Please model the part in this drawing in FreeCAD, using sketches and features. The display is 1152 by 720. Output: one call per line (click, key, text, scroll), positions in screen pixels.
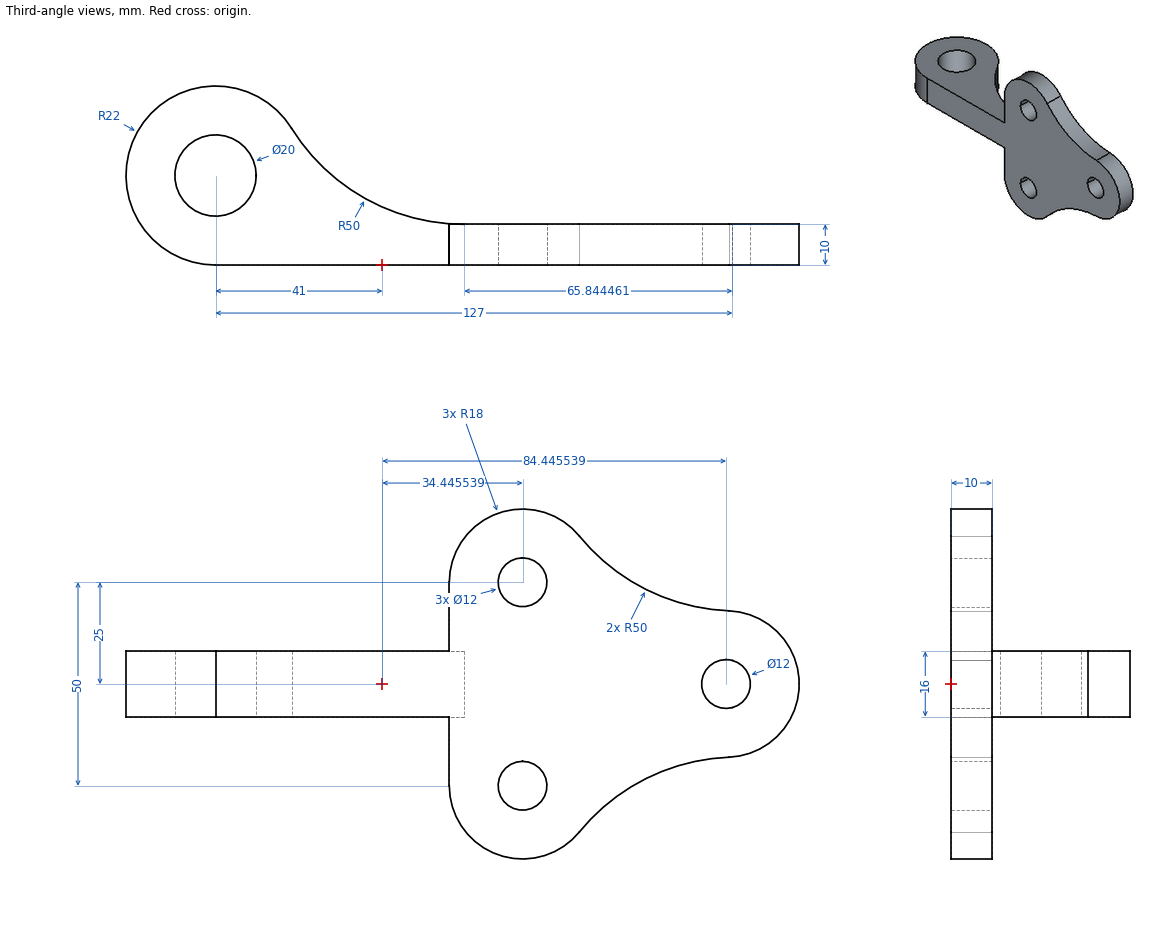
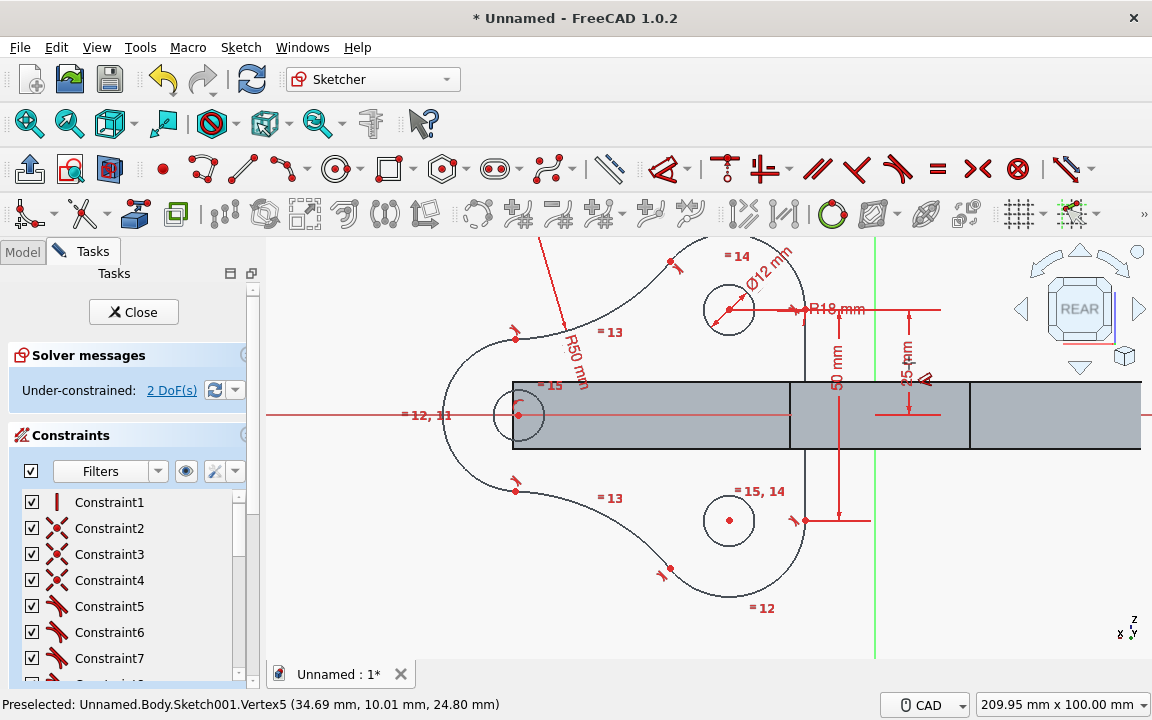
click(729, 310)
click(853, 276)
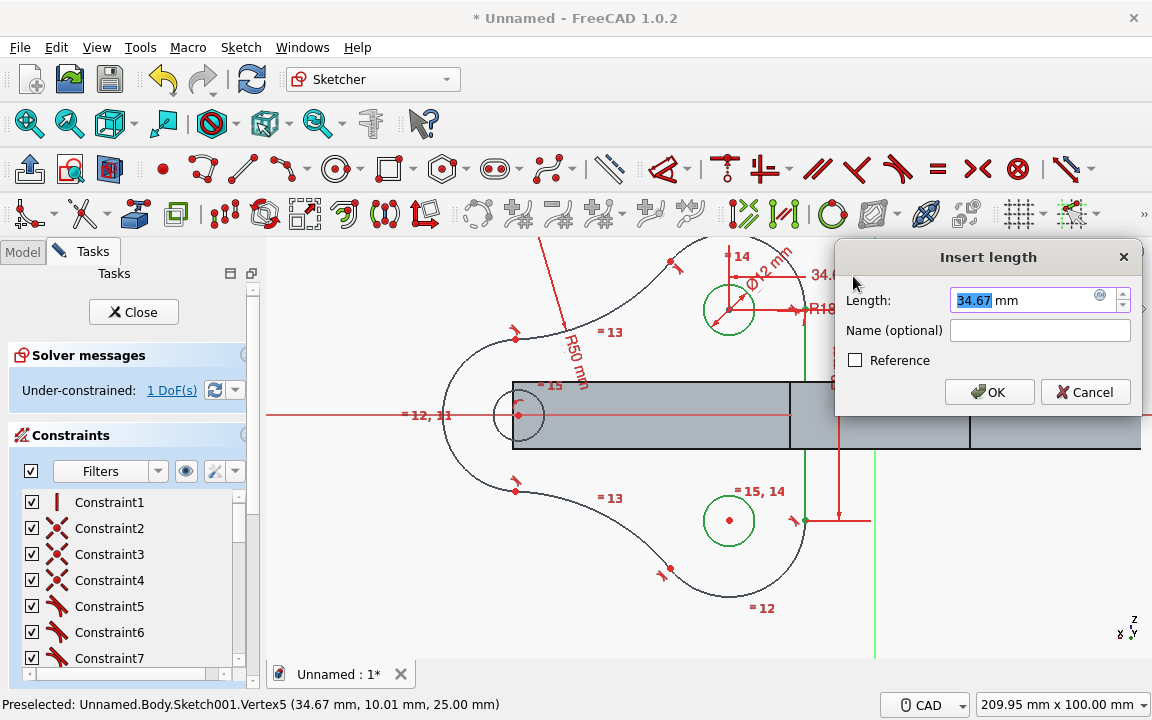
text(34.445539)
key(Return)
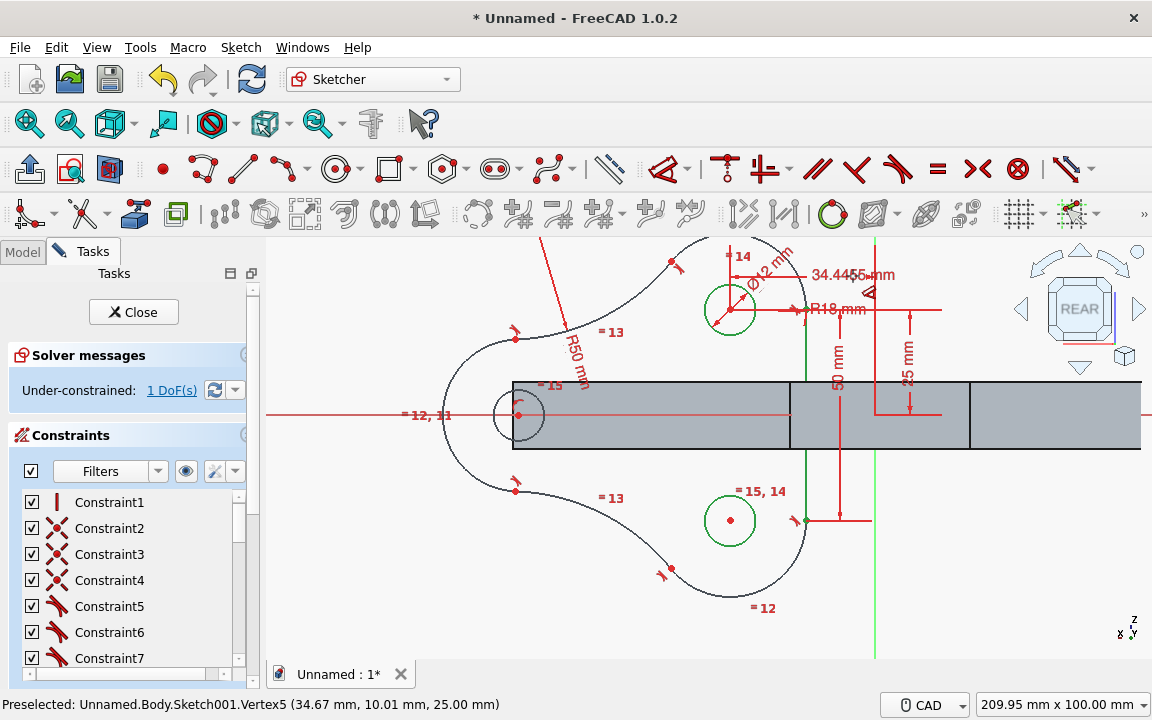
click(519, 415)
click(697, 449)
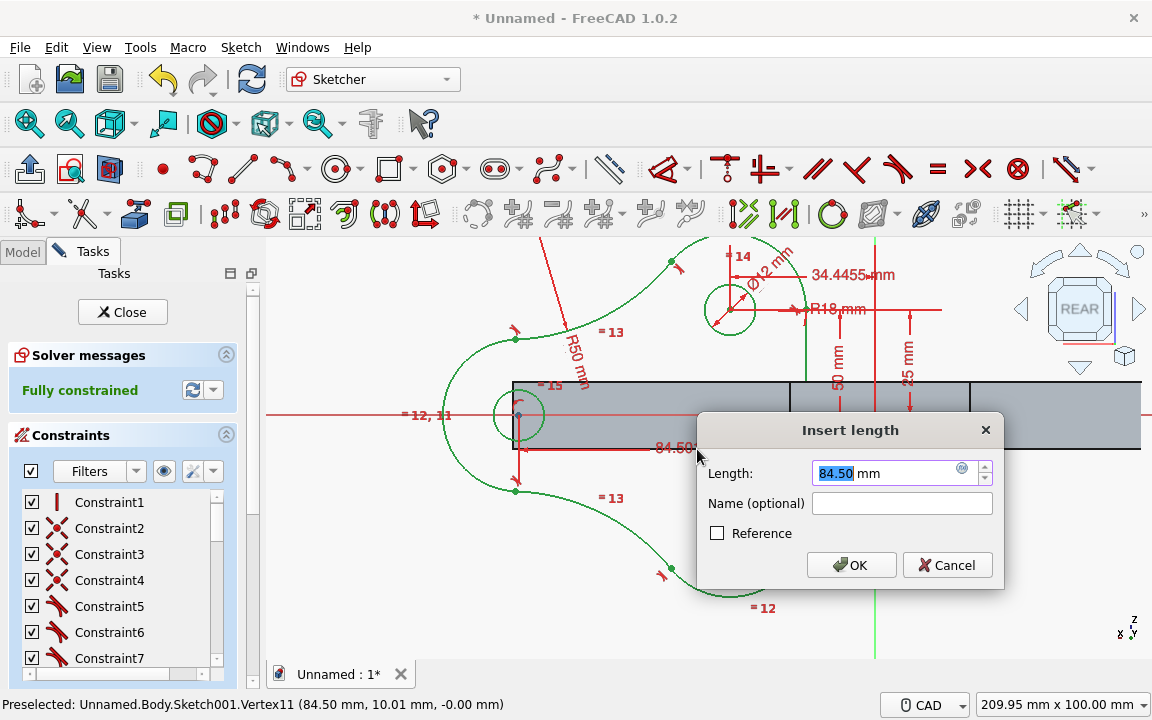
text(84.445539)
key(Return)
key(Escape)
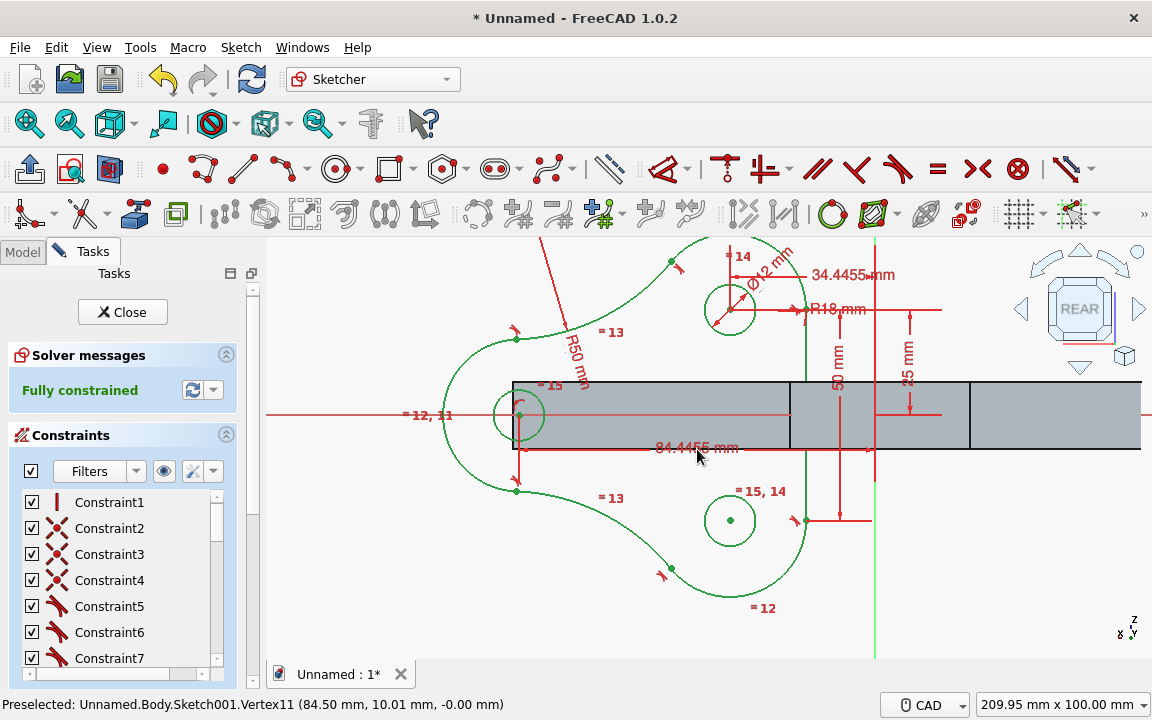
click(123, 312)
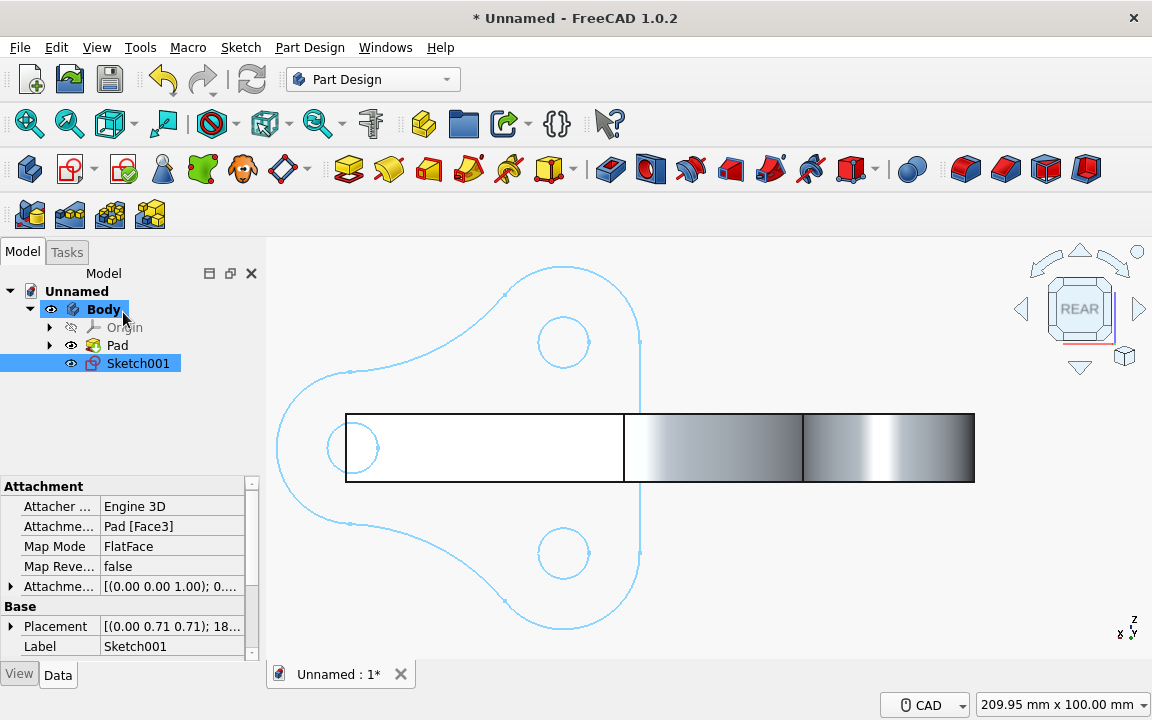
click(350, 170)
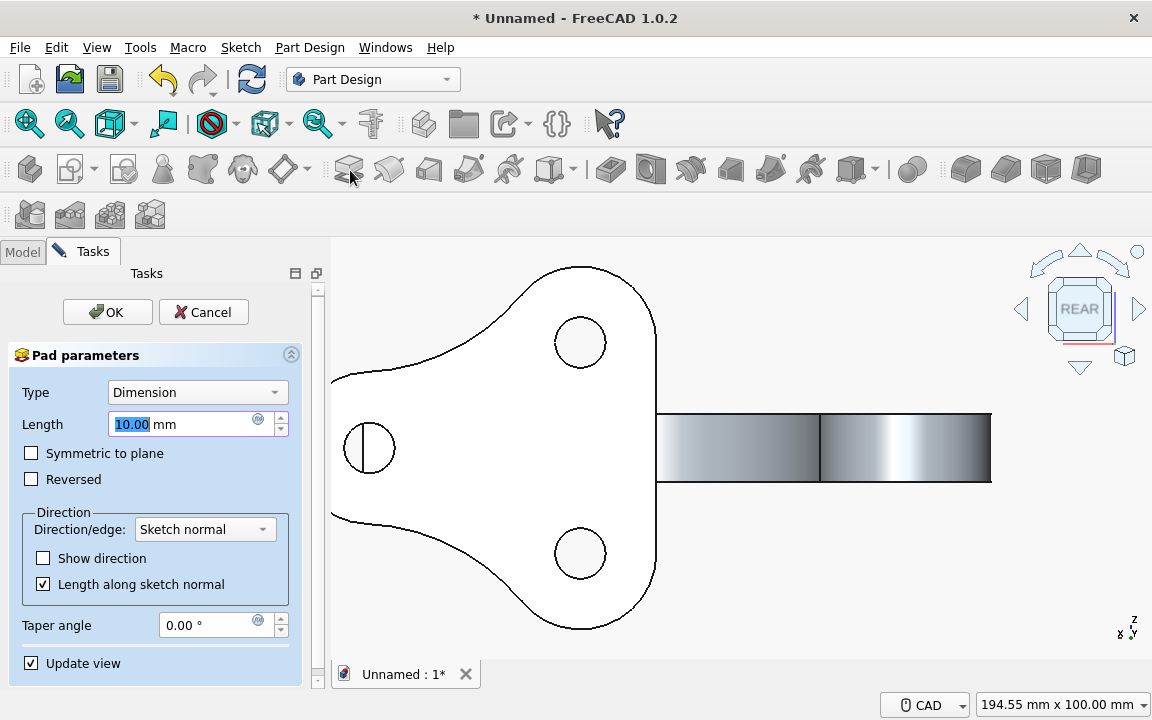
text(10)
key(Tab)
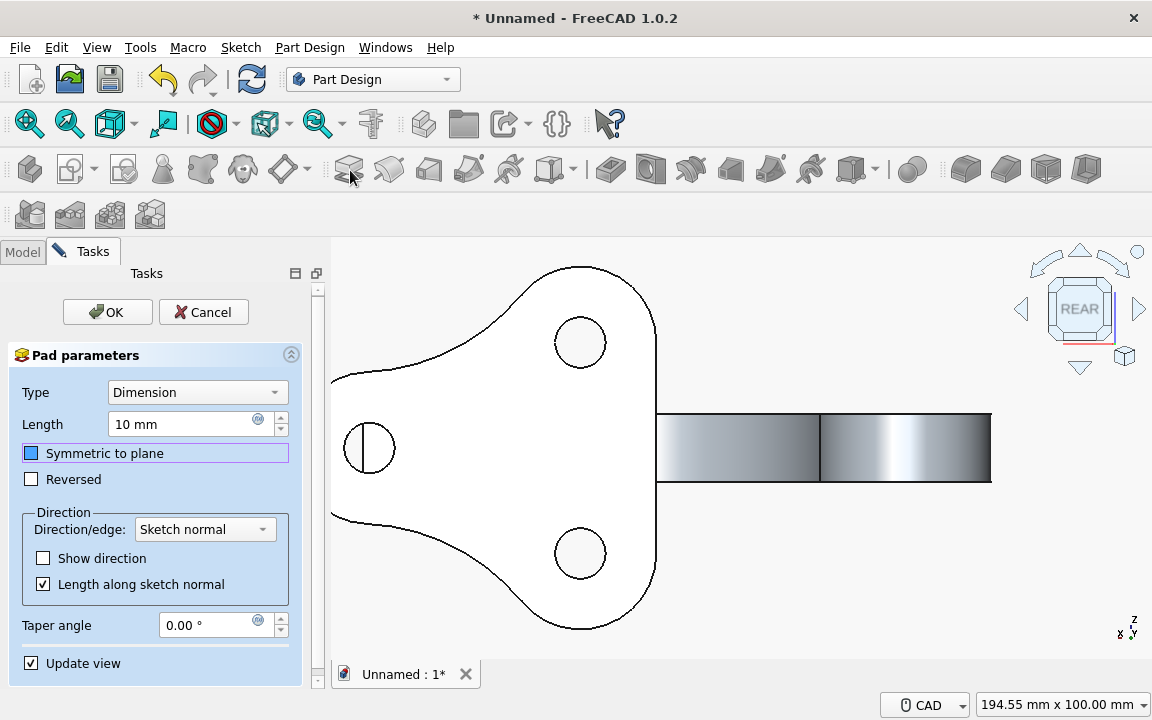
click(30, 479)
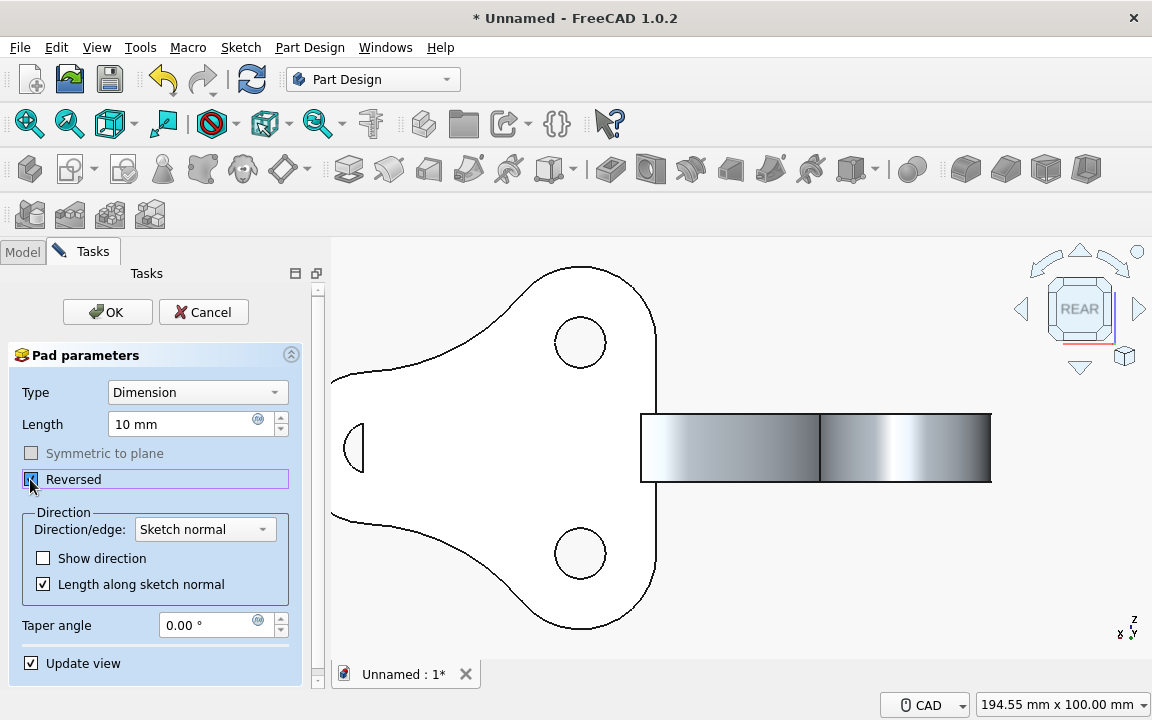
click(108, 312)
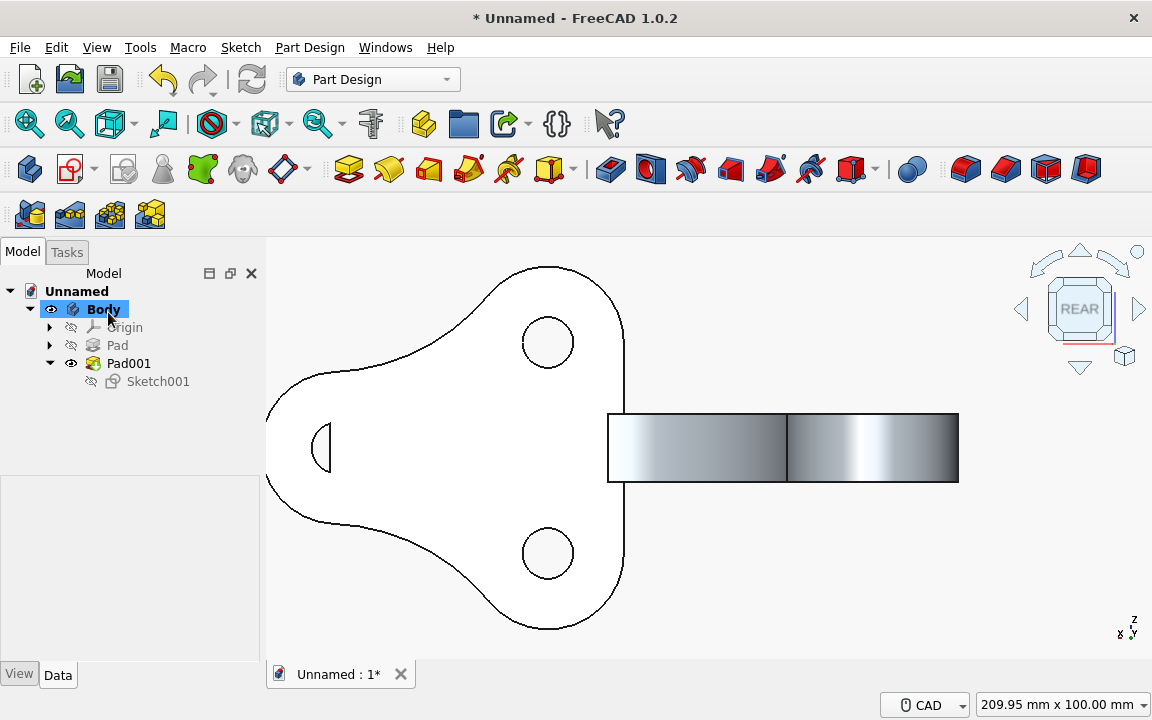
click(30, 124)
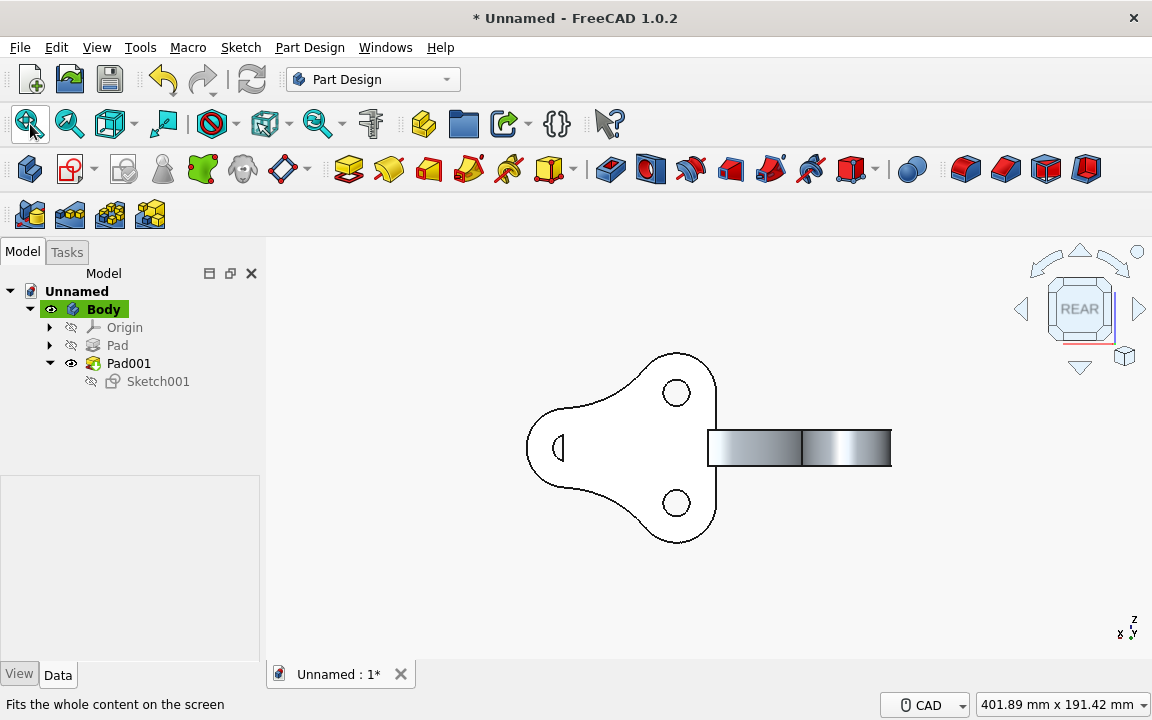
click(621, 447)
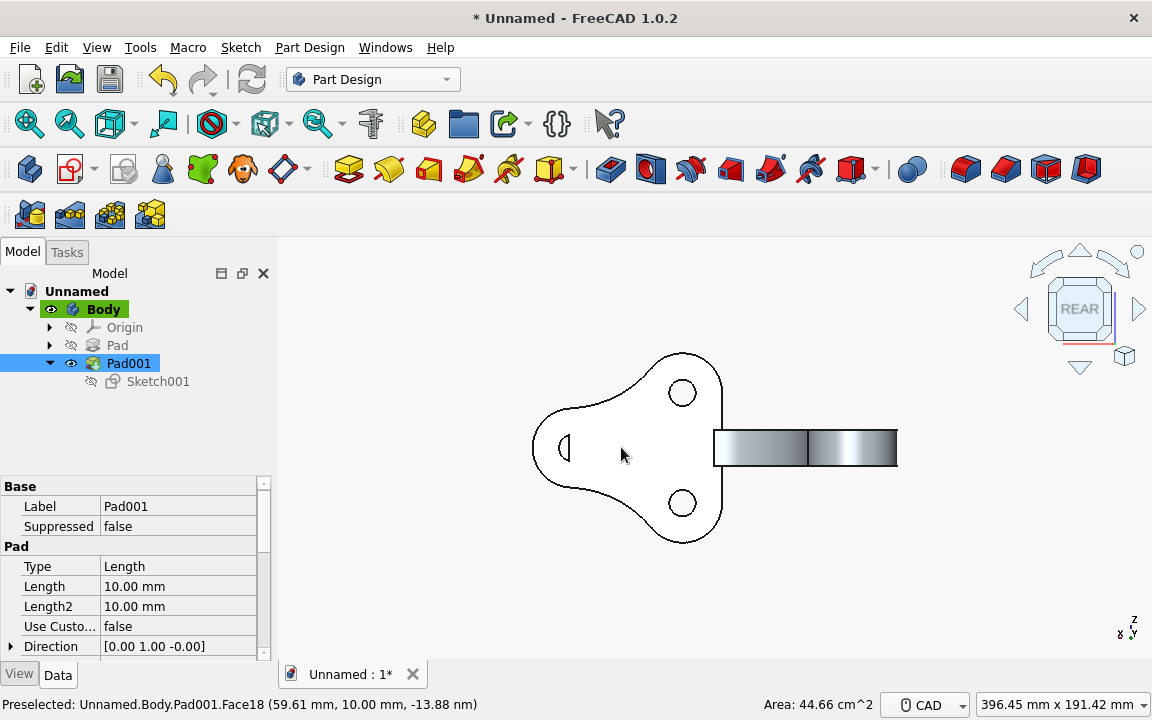
click(70, 170)